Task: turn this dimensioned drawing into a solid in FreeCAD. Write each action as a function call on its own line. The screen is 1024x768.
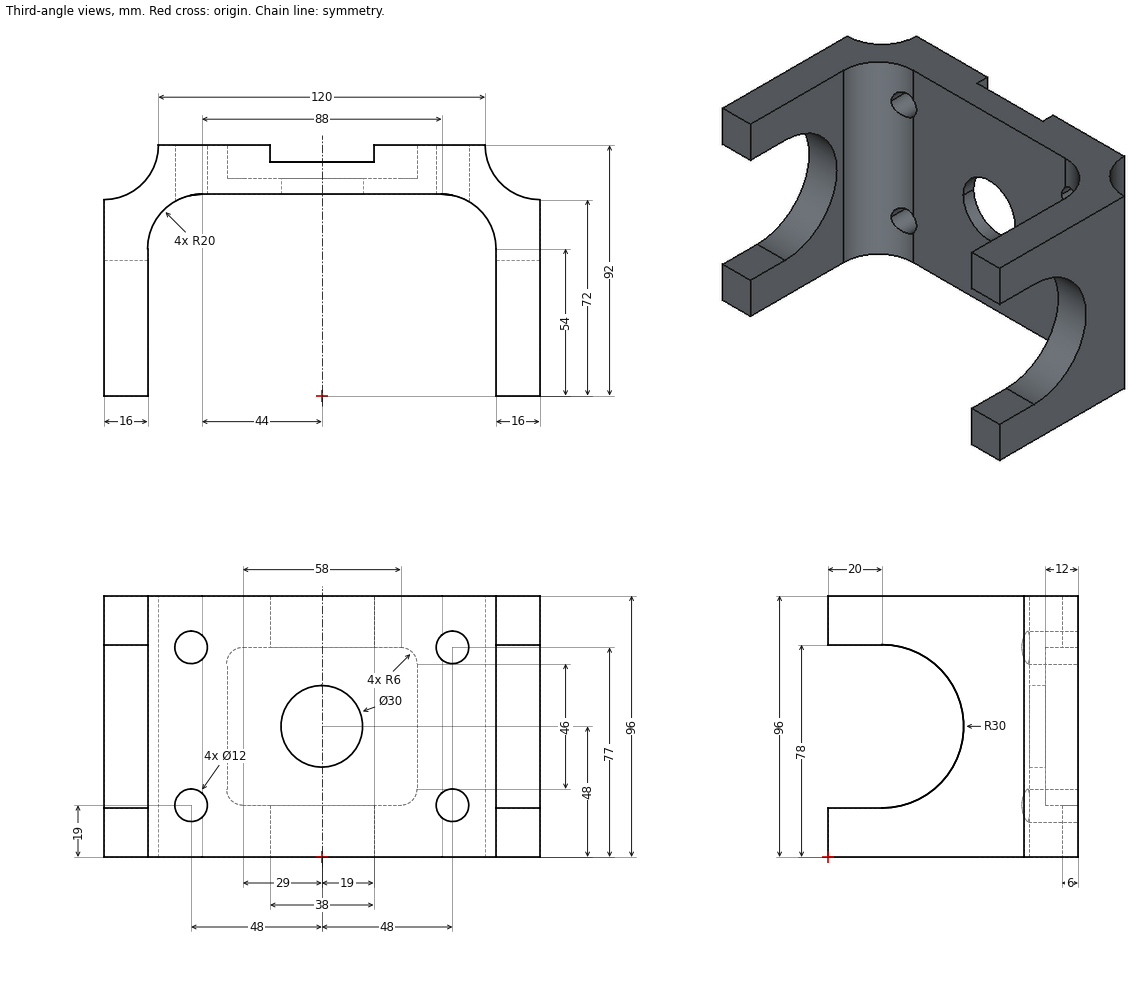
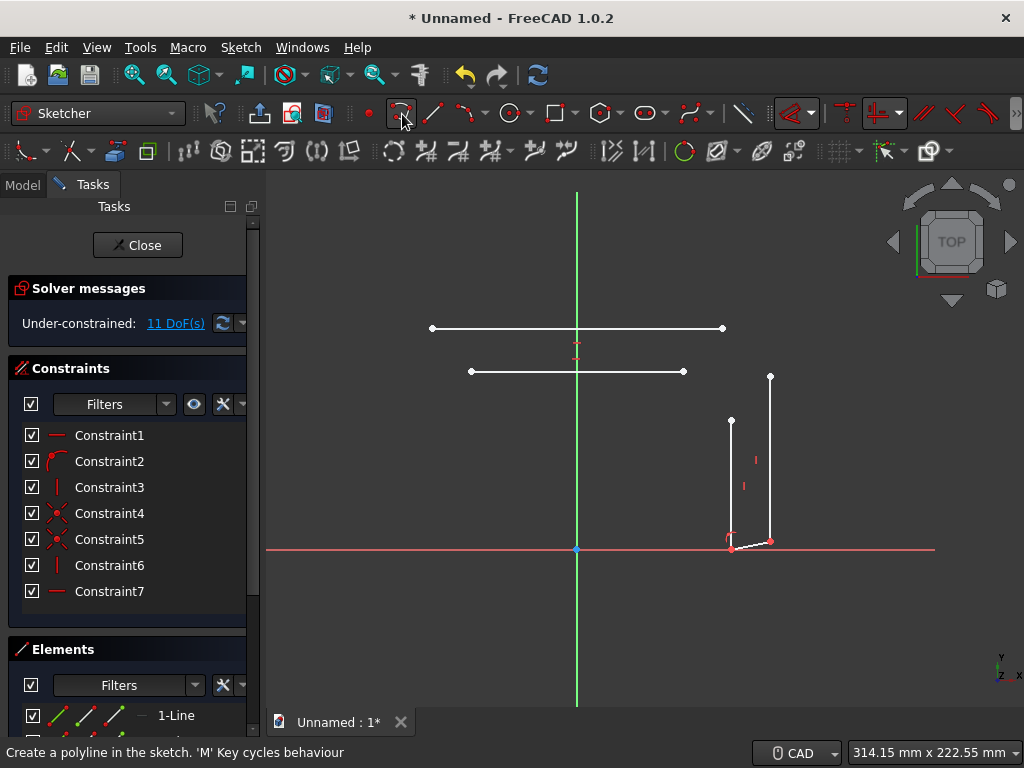
click(384, 376)
click(384, 550)
click(422, 541)
click(422, 420)
right_click(422, 420)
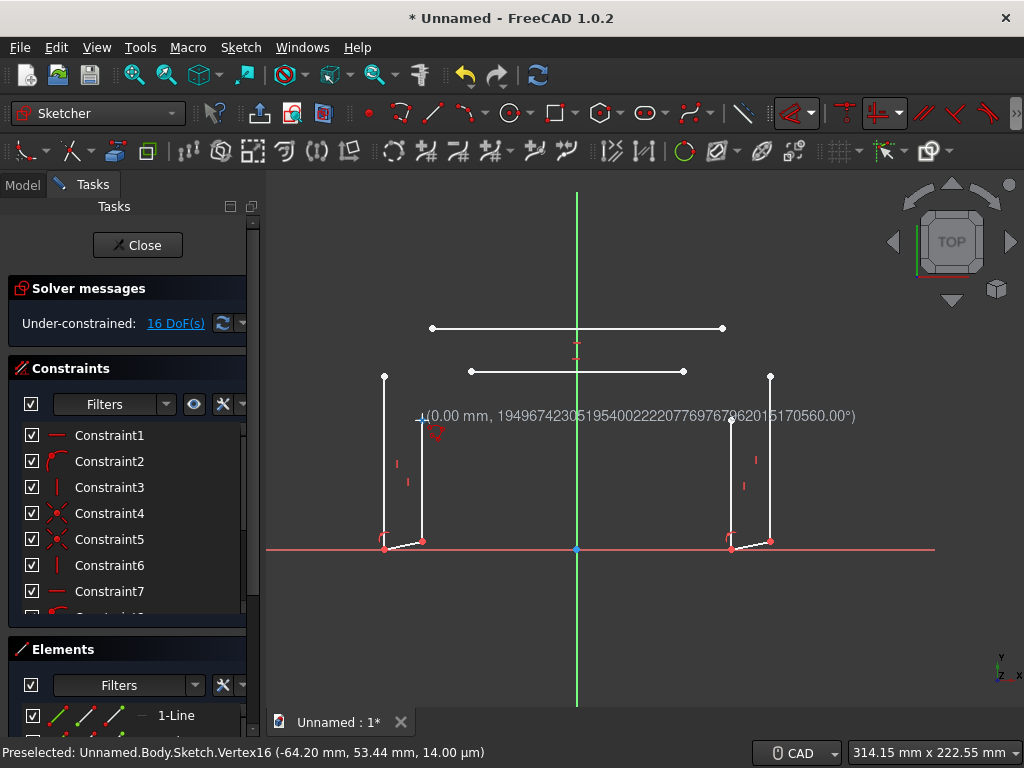
click(466, 114)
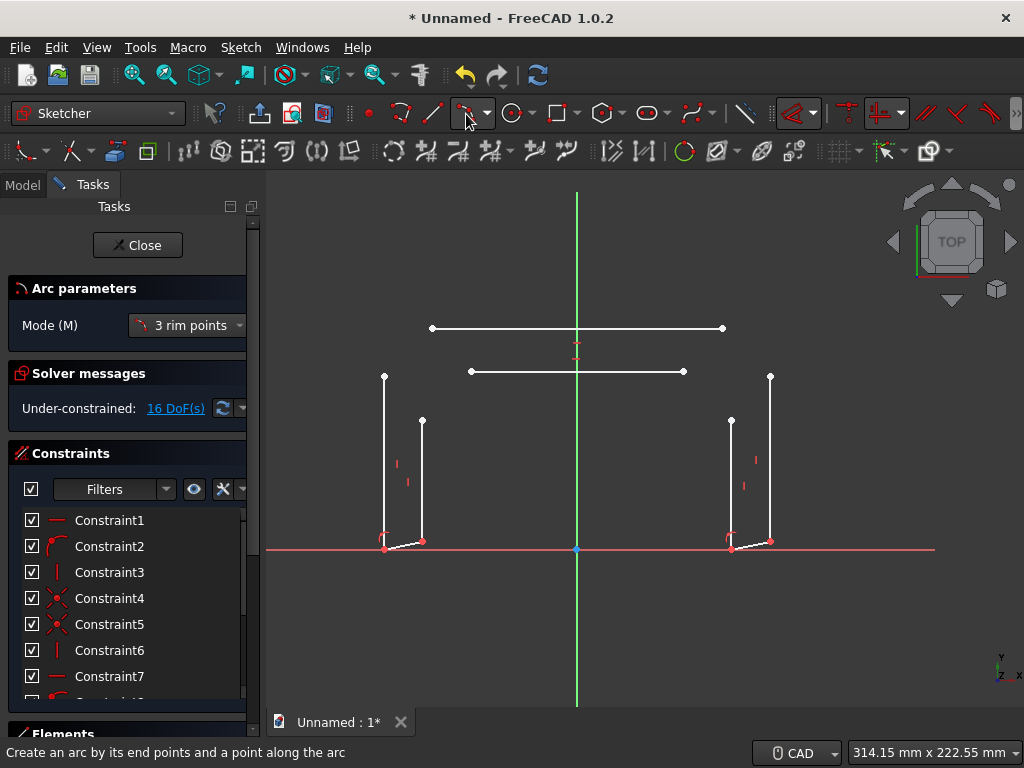
click(683, 372)
click(731, 421)
click(717, 386)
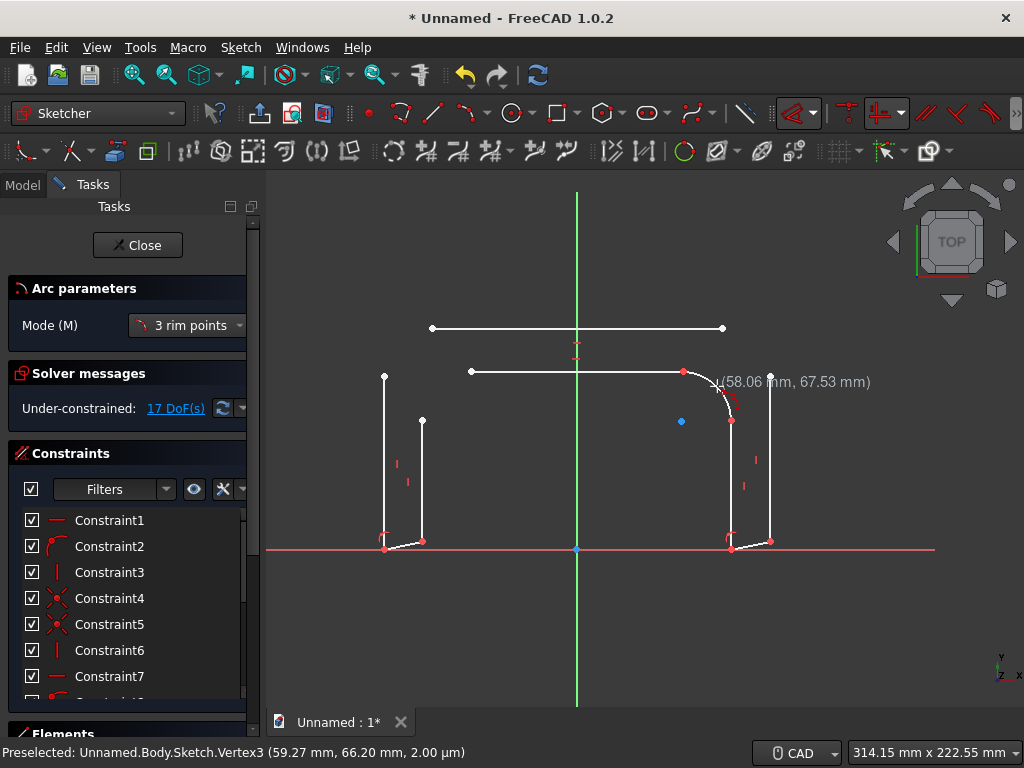
click(770, 377)
click(722, 329)
click(736, 362)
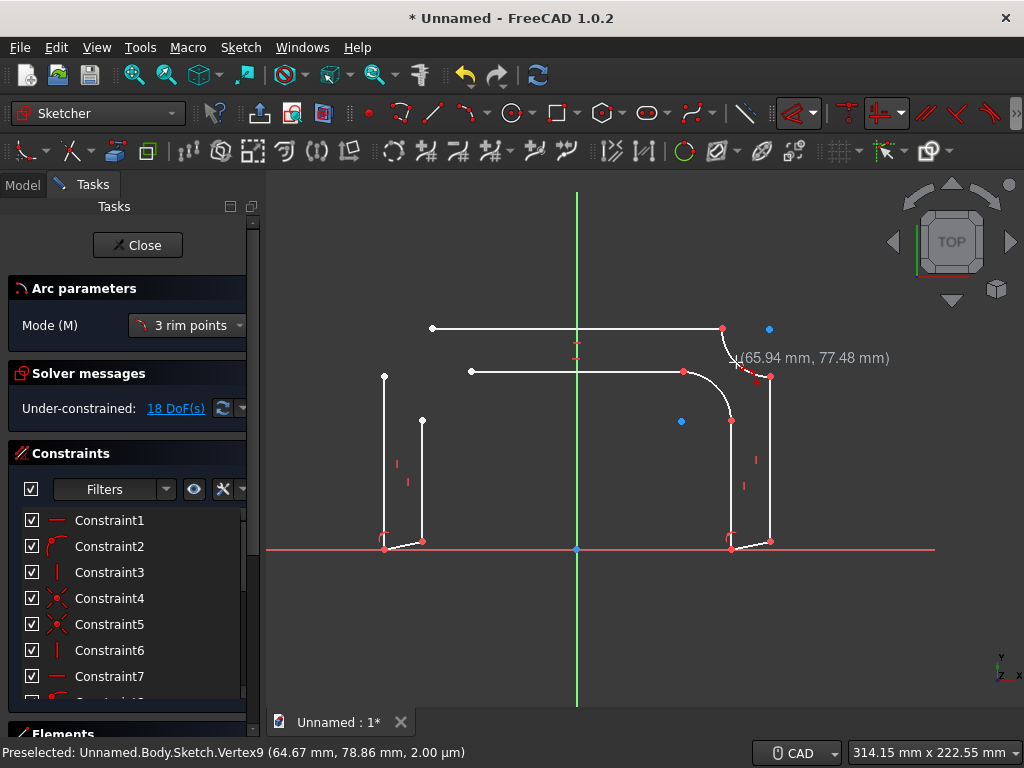
click(432, 329)
click(384, 377)
click(418, 362)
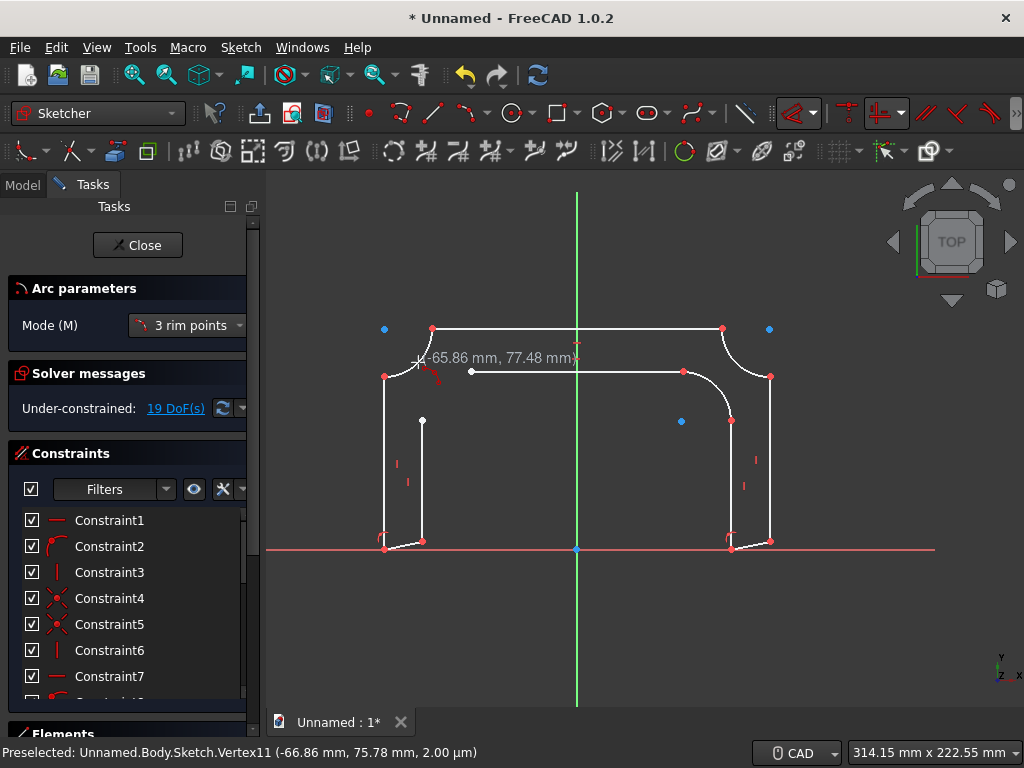
click(422, 421)
click(471, 372)
click(437, 386)
key(Escape)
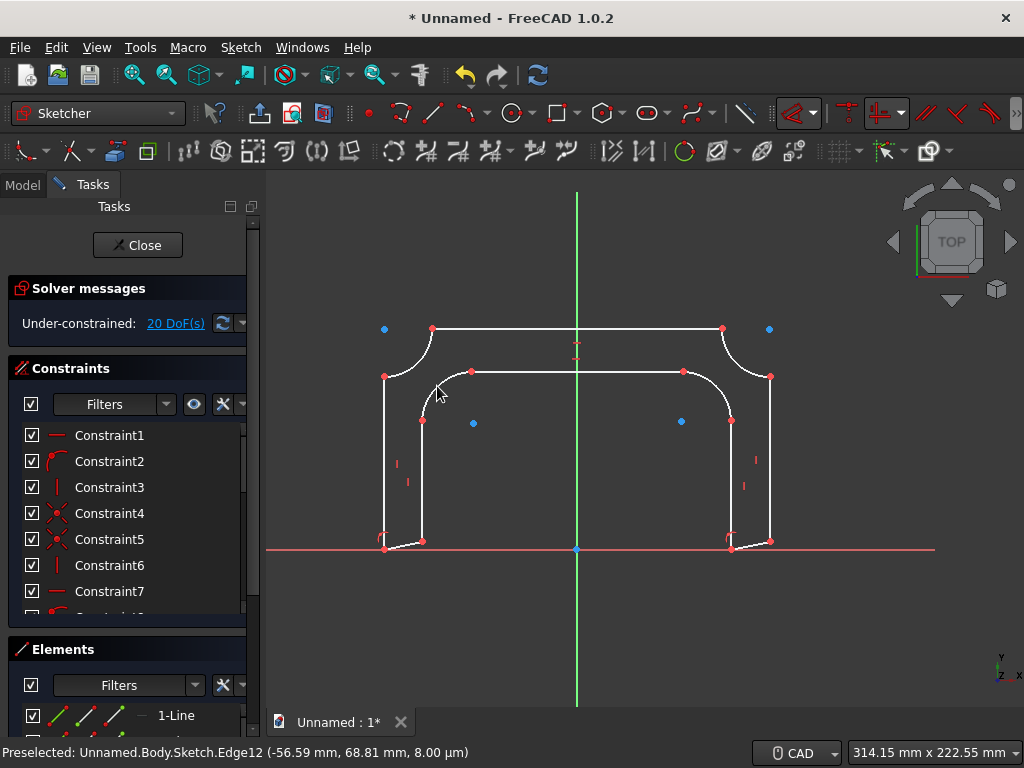
click(535, 372)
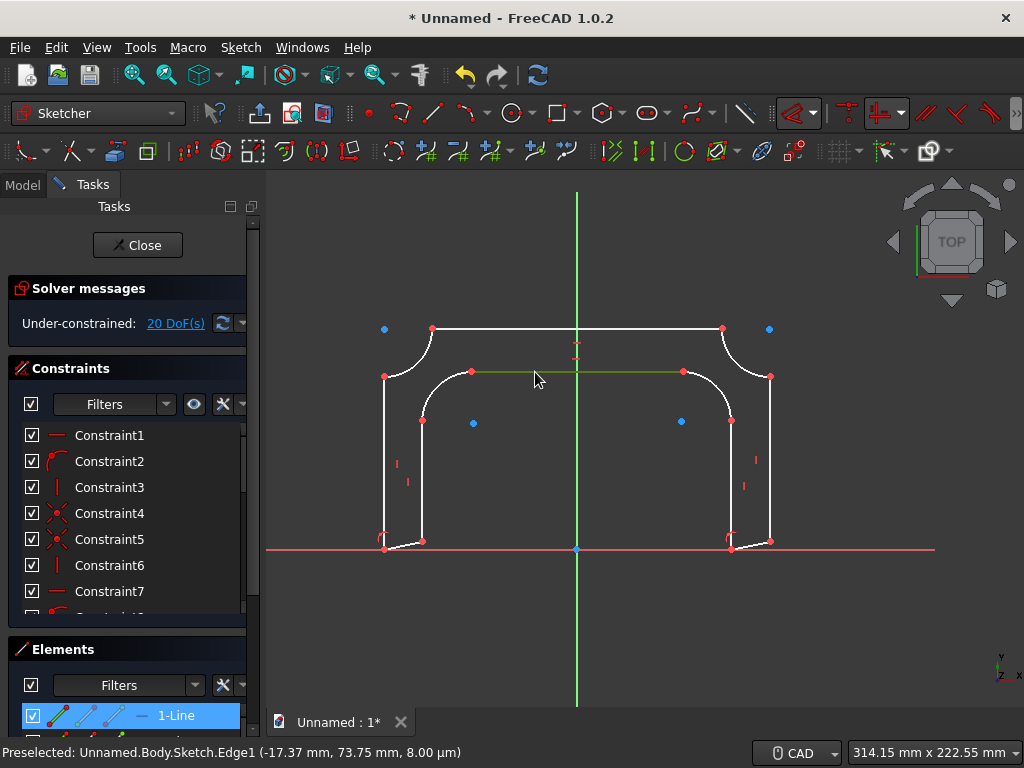
click(726, 399)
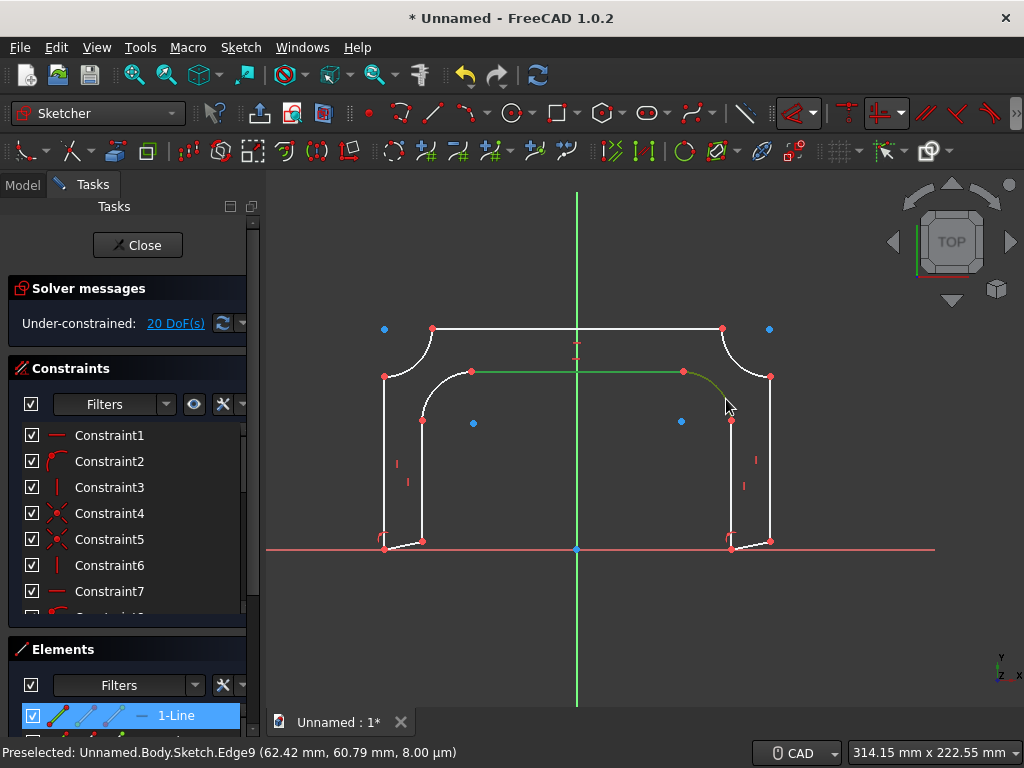
click(990, 114)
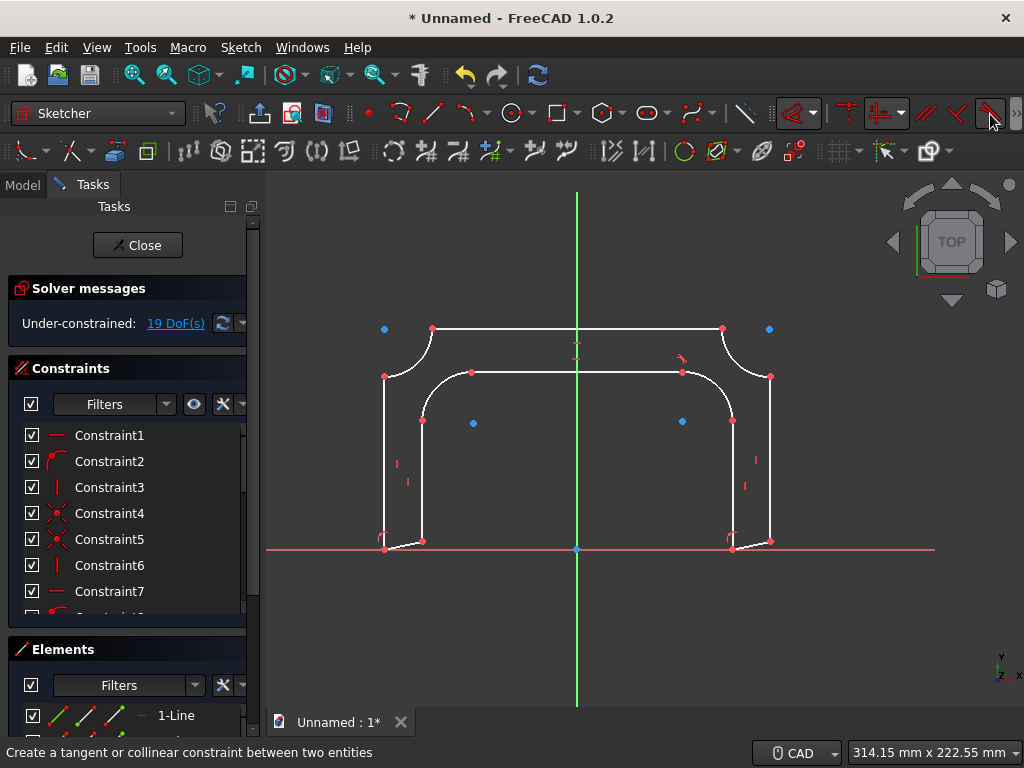
click(535, 372)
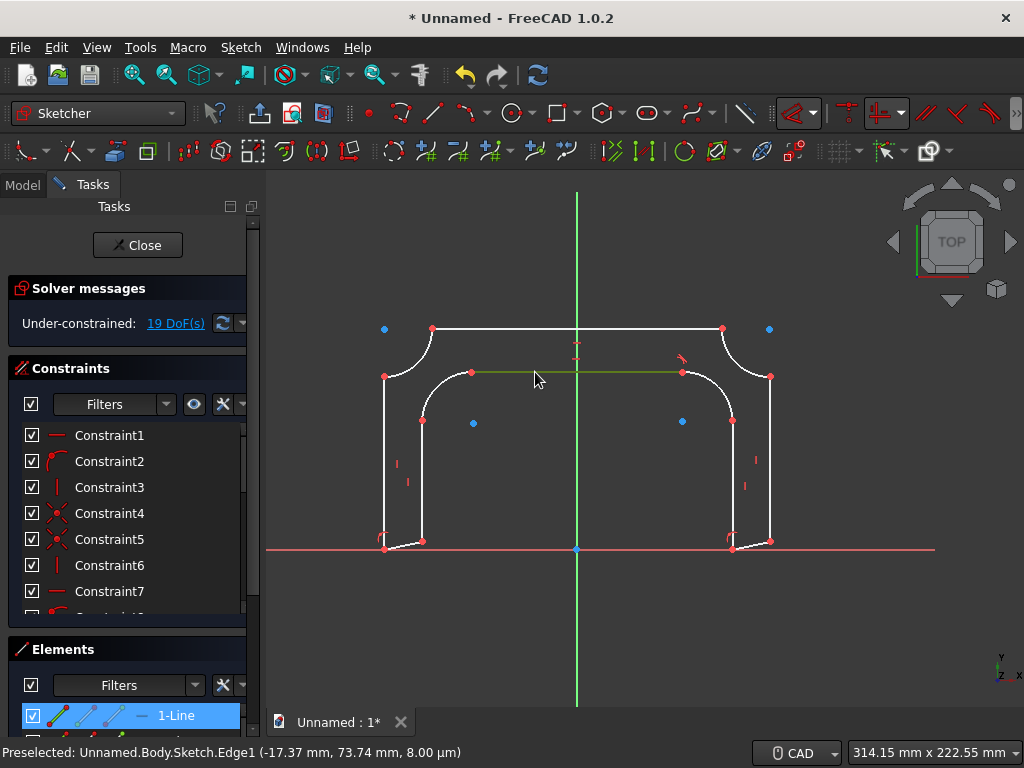
click(449, 378)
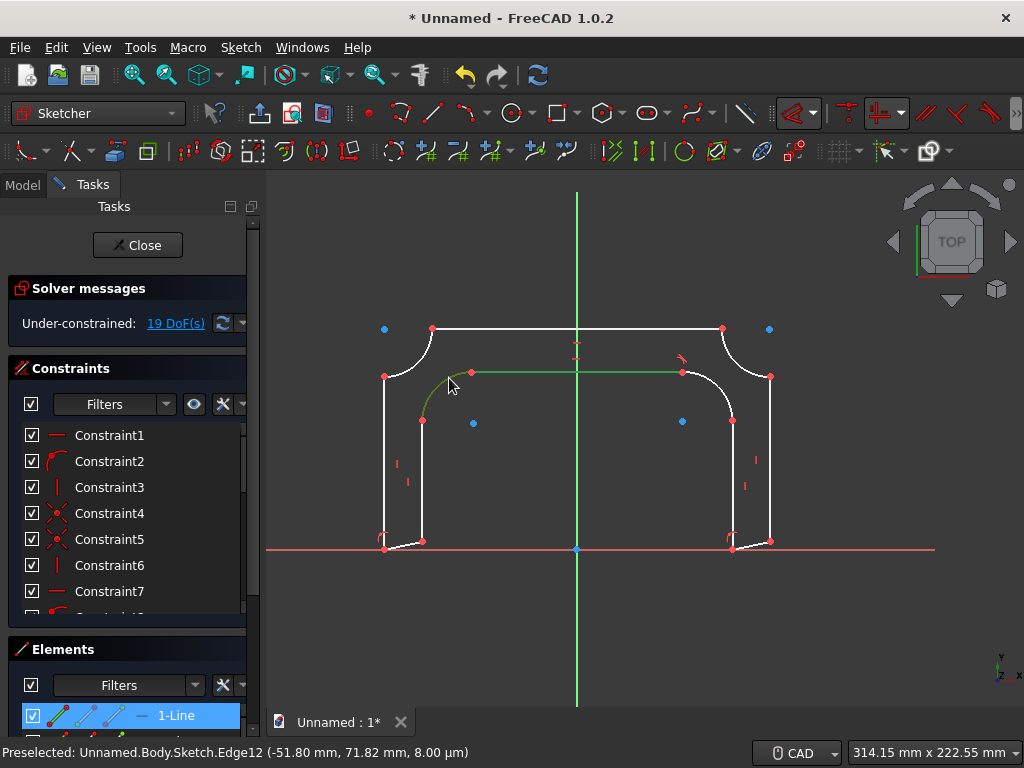
click(990, 114)